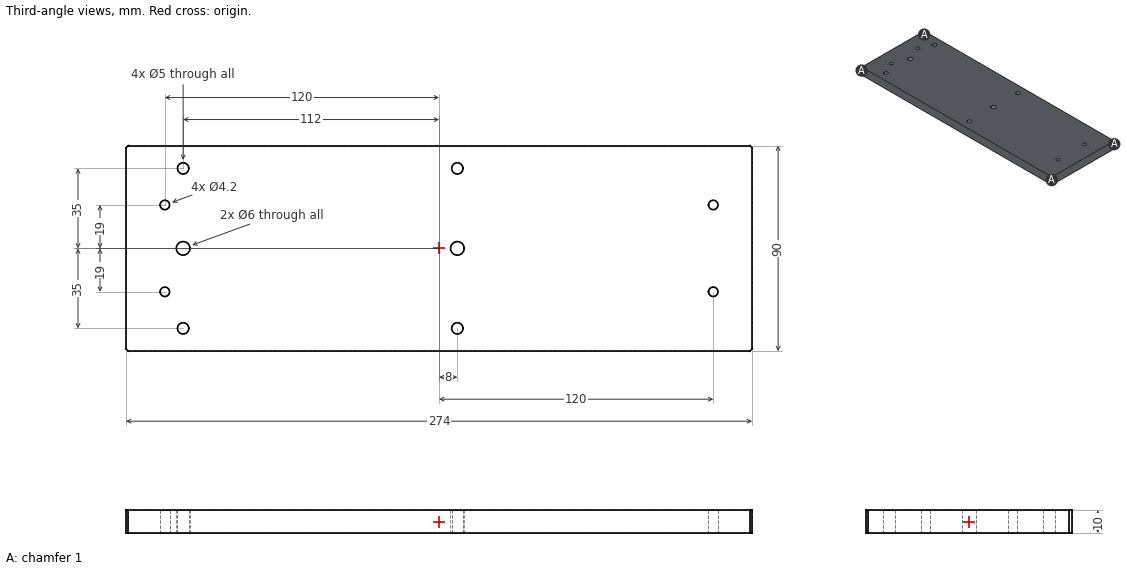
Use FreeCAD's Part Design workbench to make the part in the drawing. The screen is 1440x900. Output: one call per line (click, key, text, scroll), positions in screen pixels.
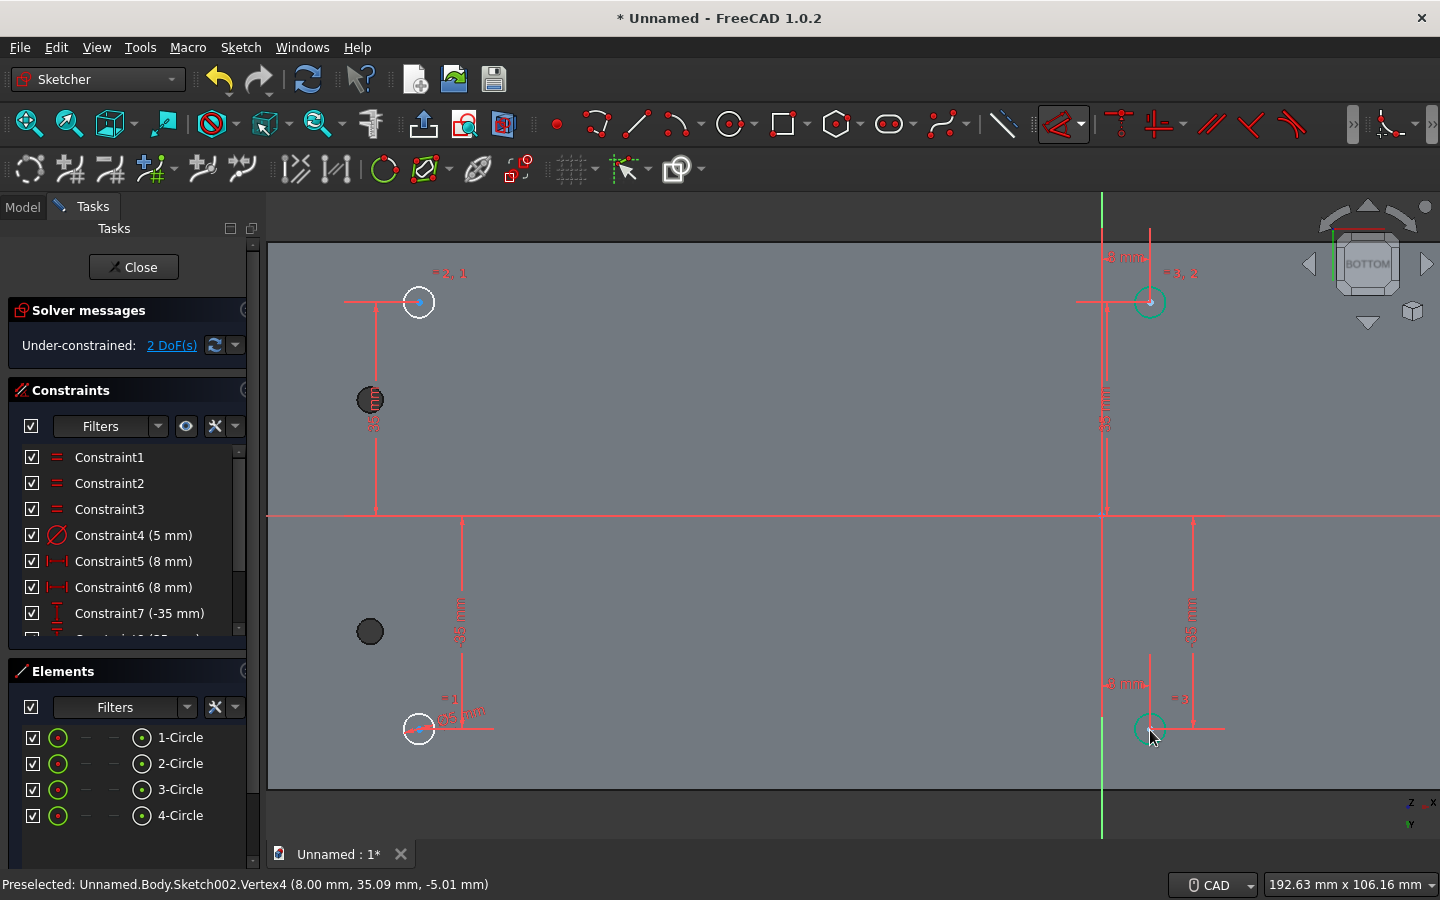
click(419, 729)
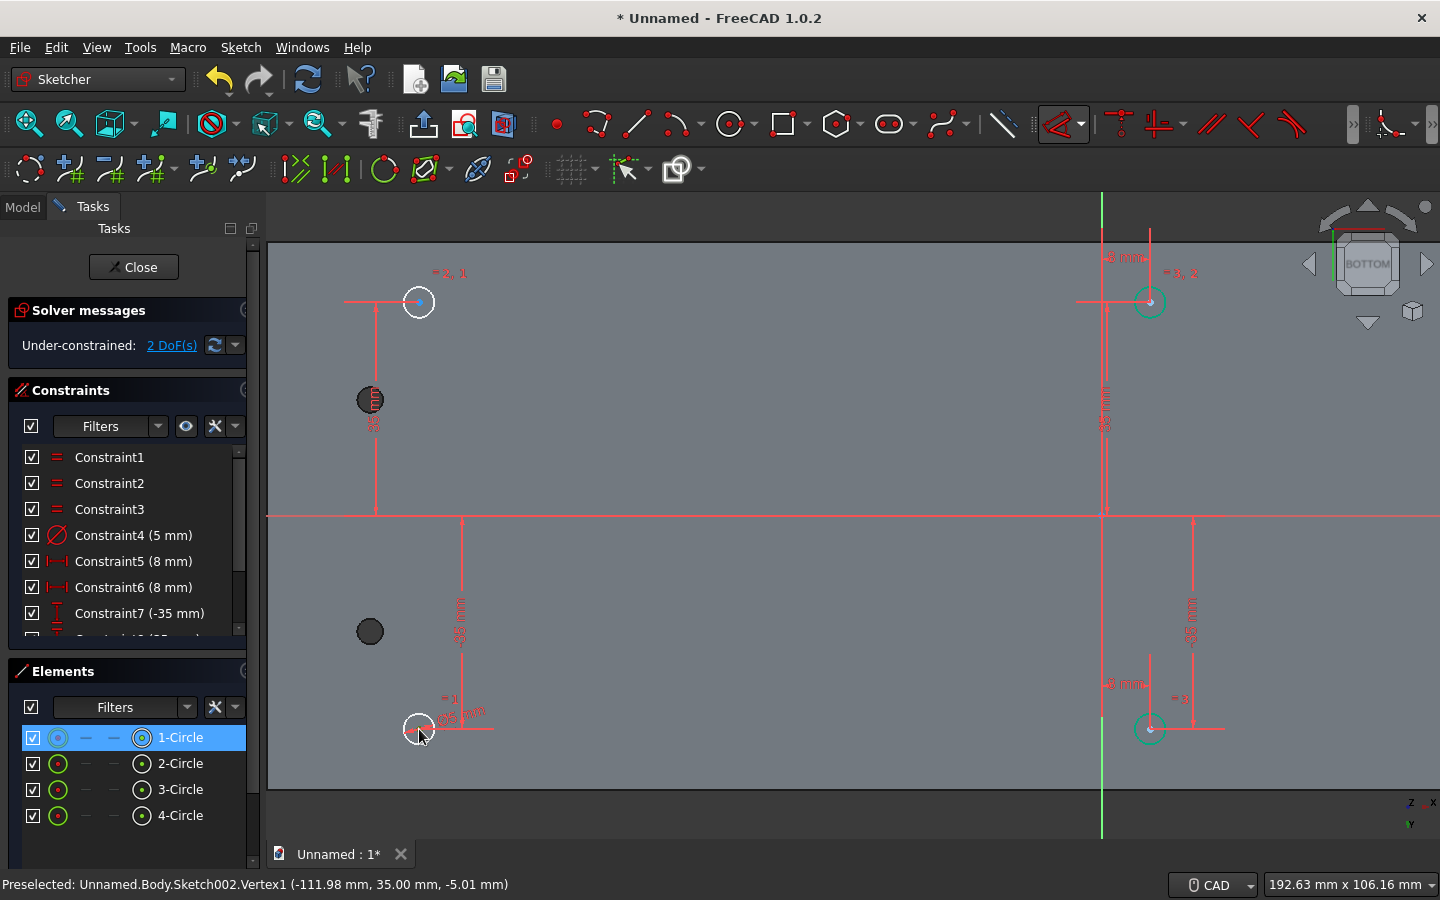
click(1084, 124)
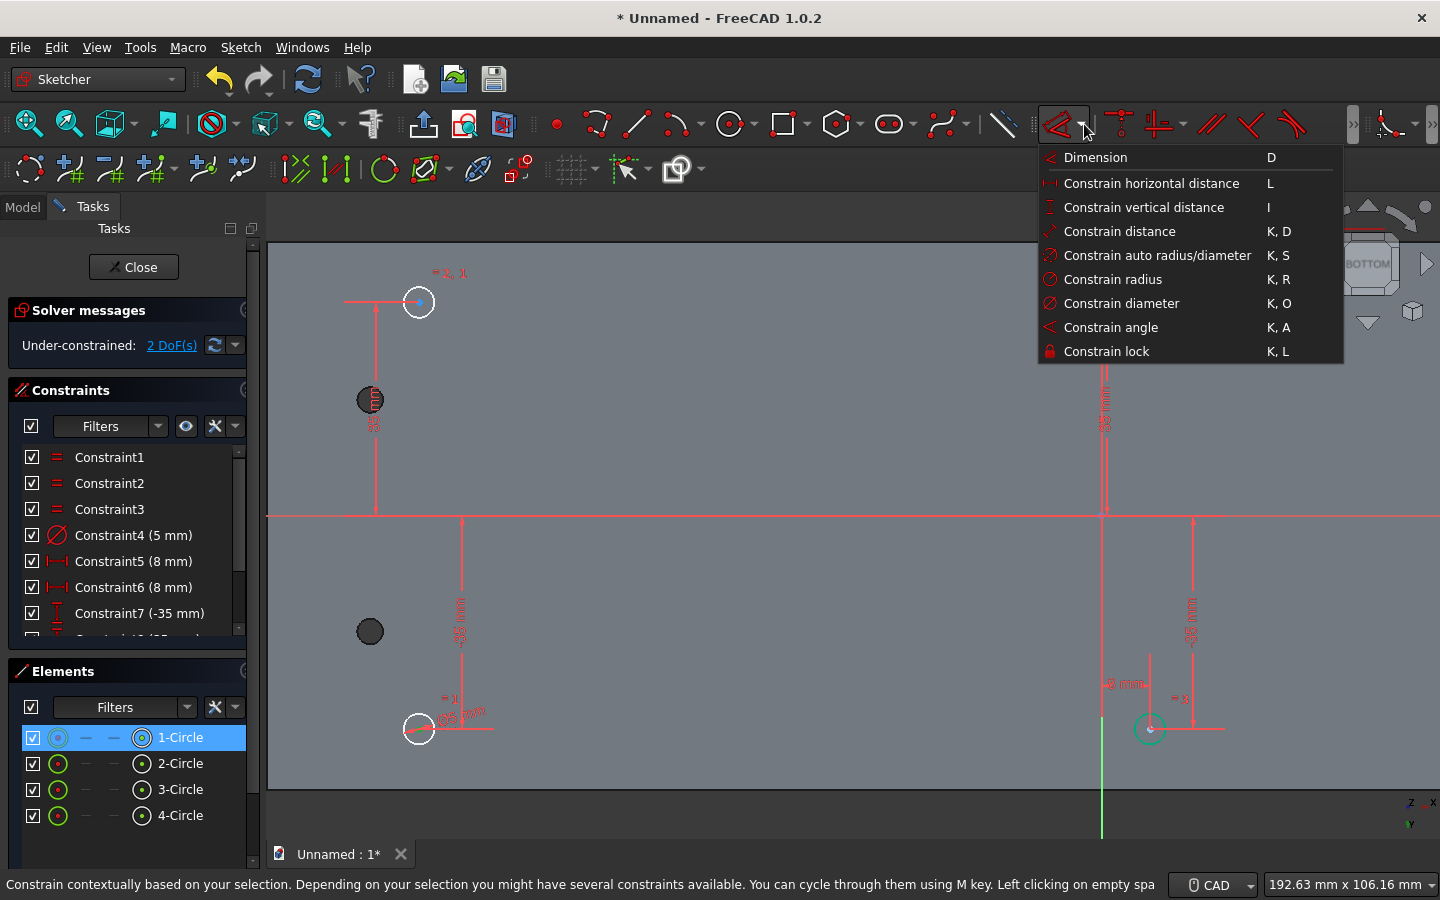
click(1191, 183)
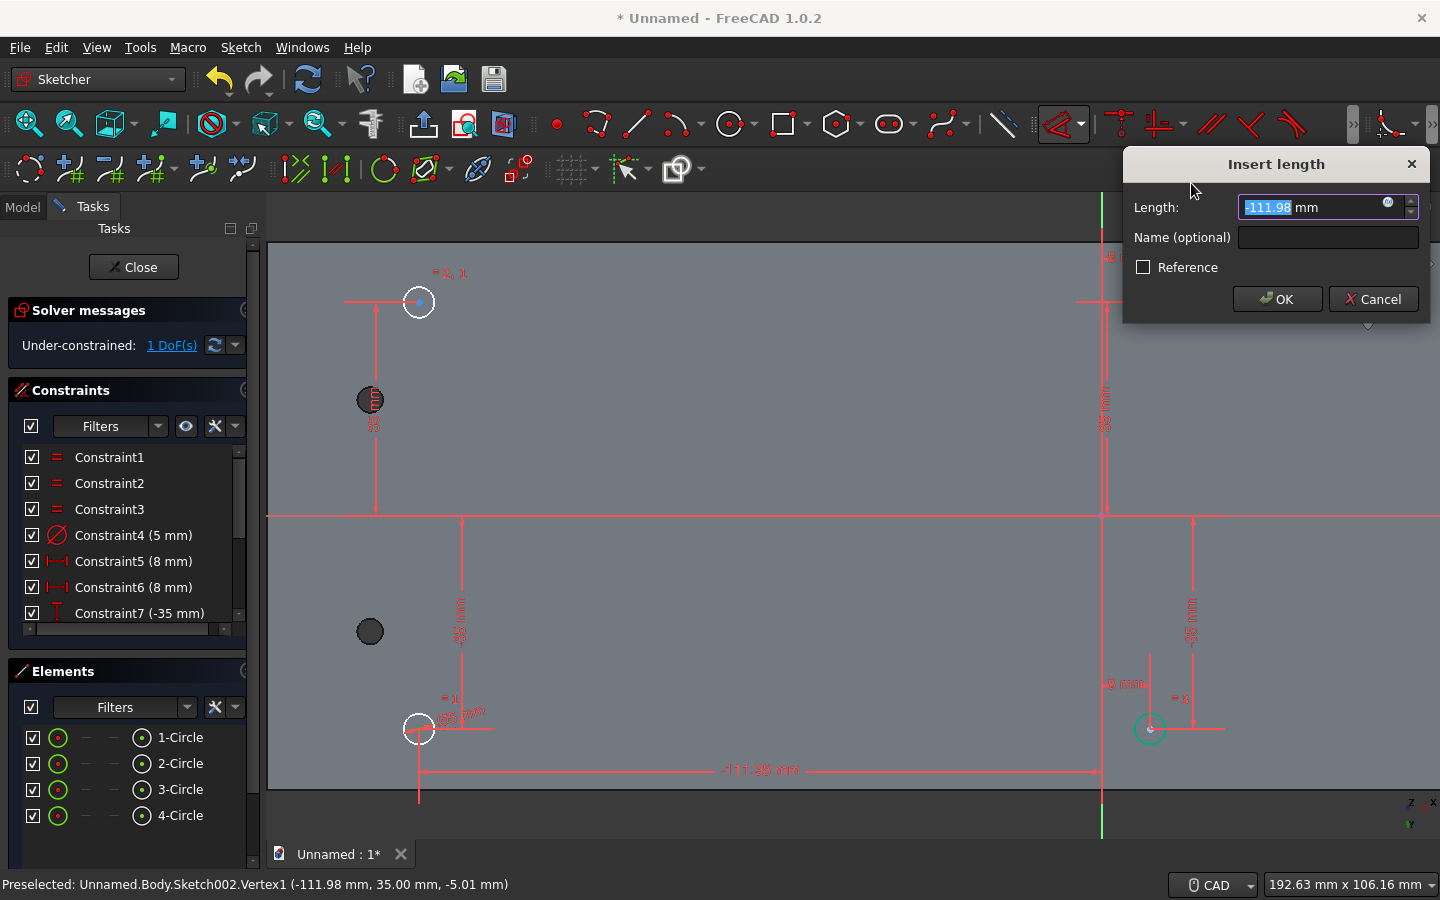
text(-112)
key(Return)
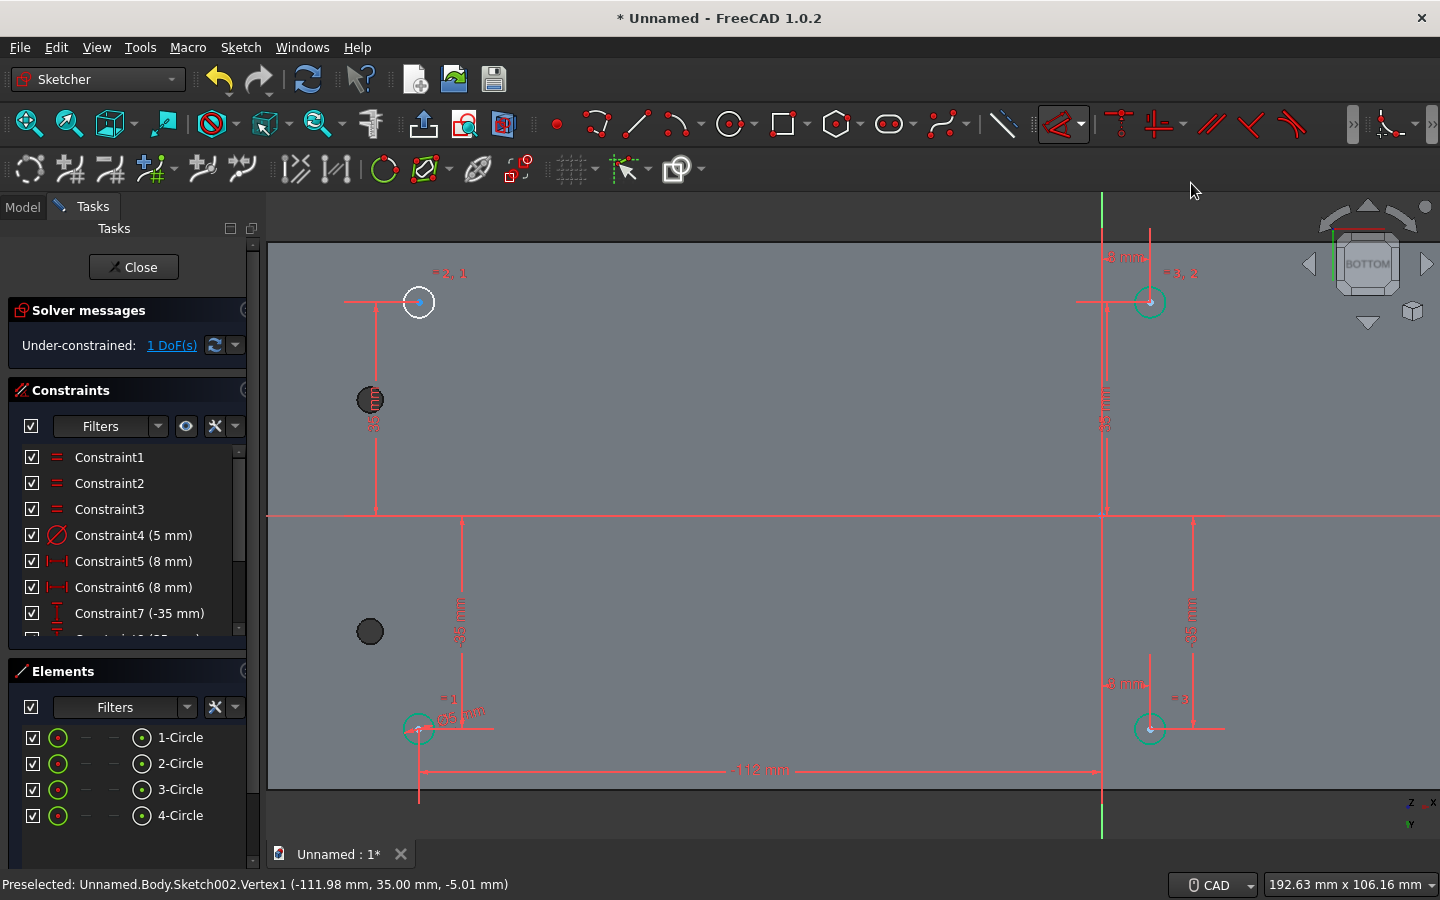
click(419, 302)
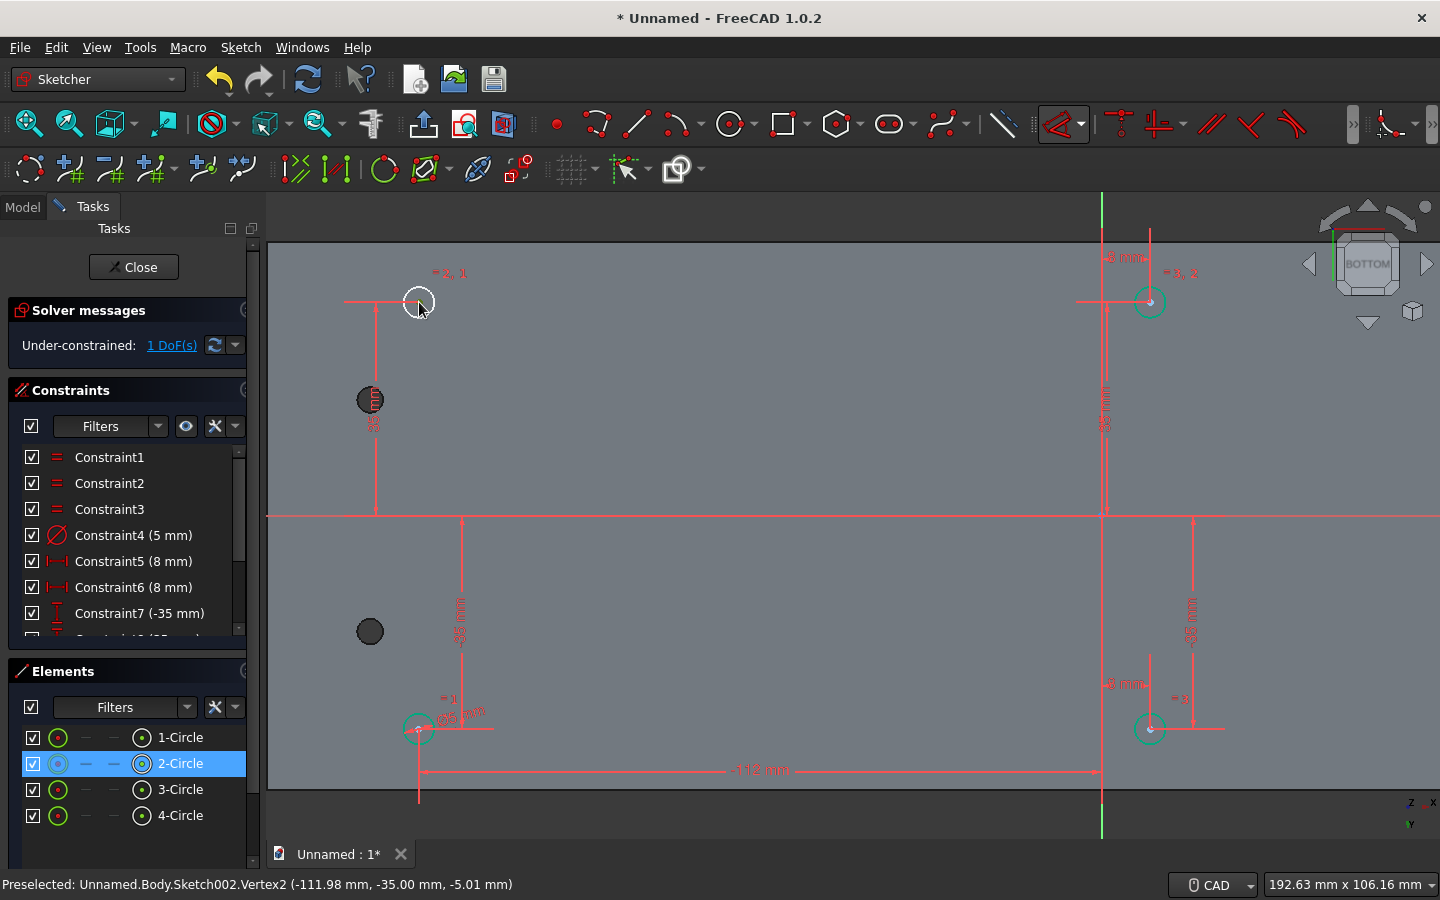
key(l)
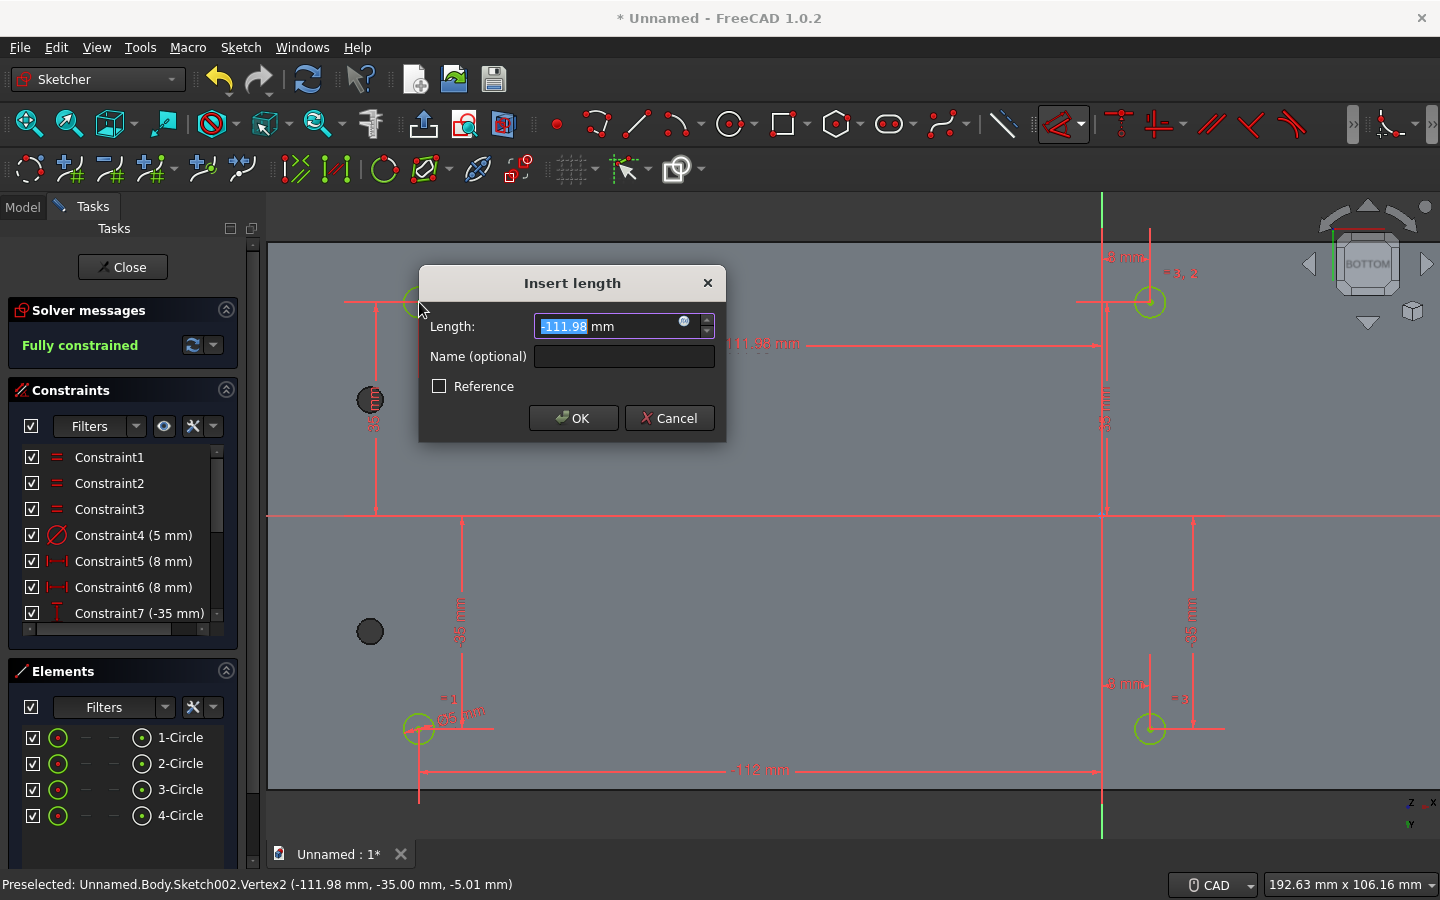
text(-112)
key(Return)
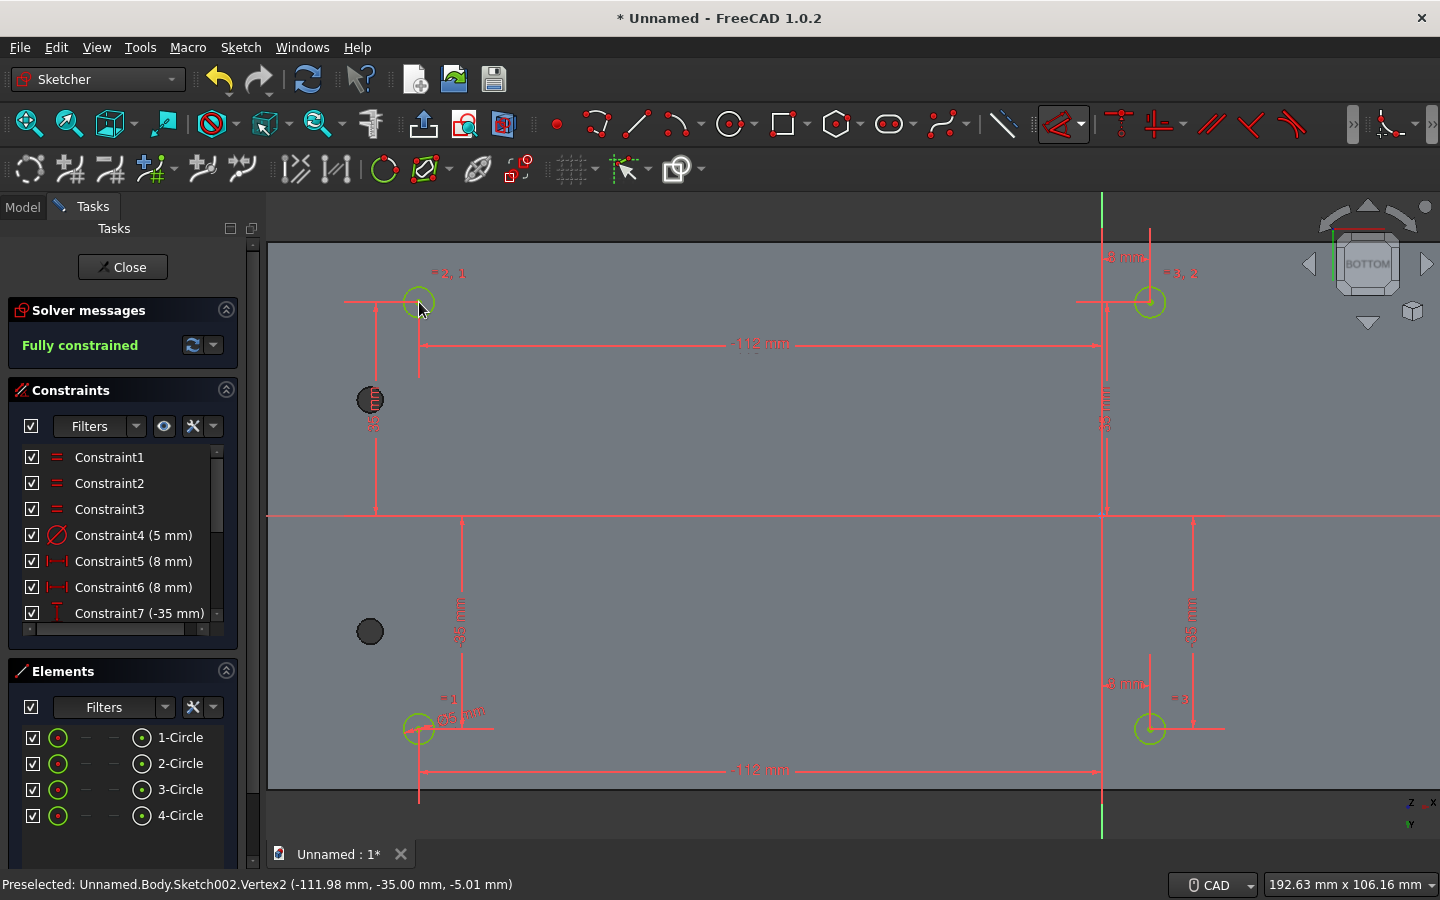
click(123, 267)